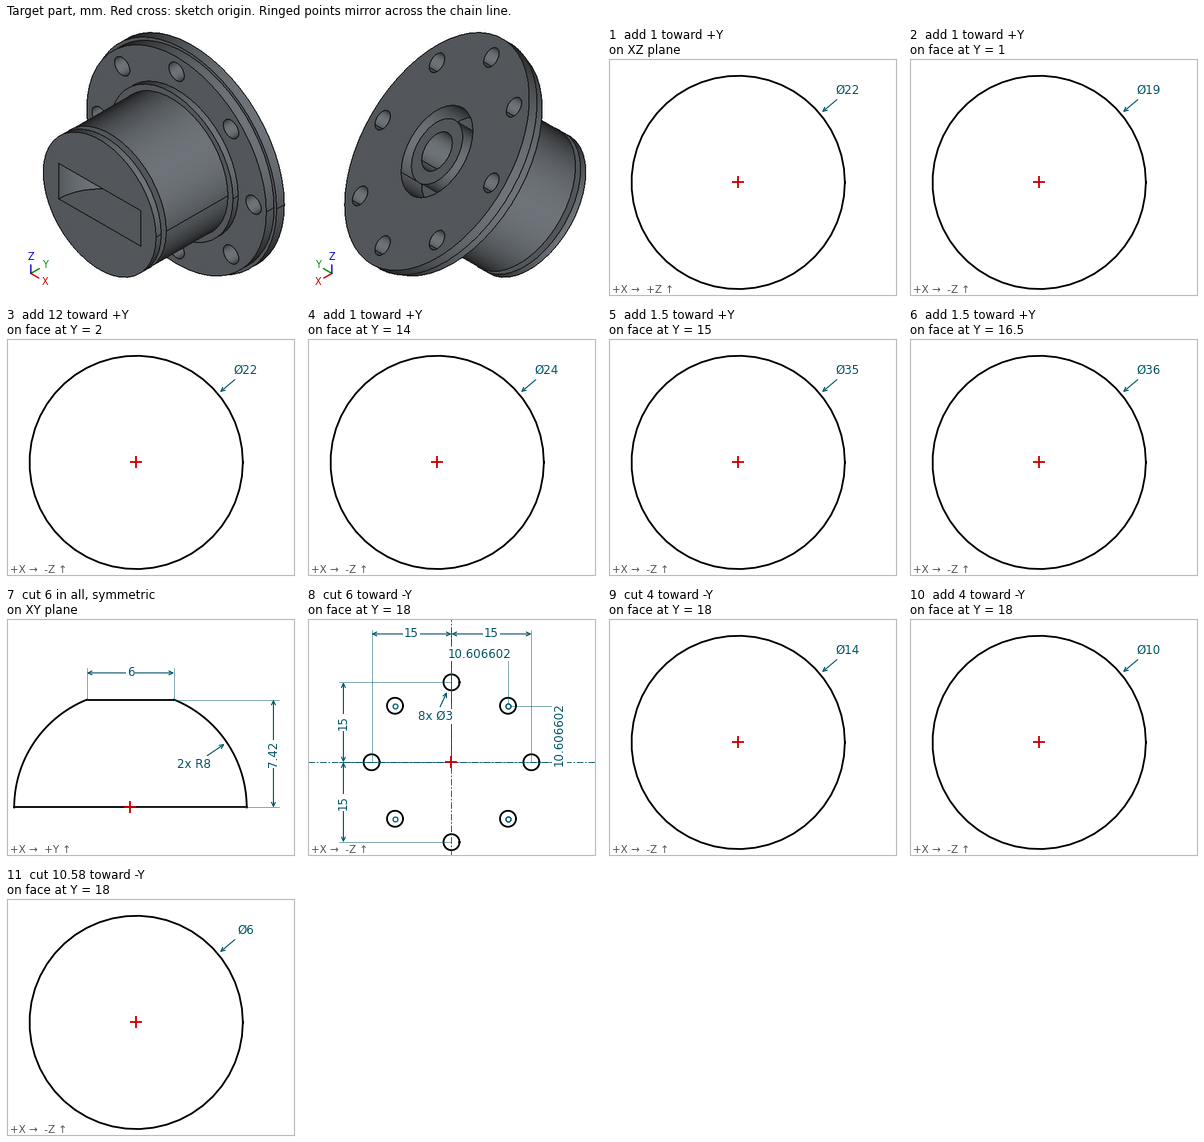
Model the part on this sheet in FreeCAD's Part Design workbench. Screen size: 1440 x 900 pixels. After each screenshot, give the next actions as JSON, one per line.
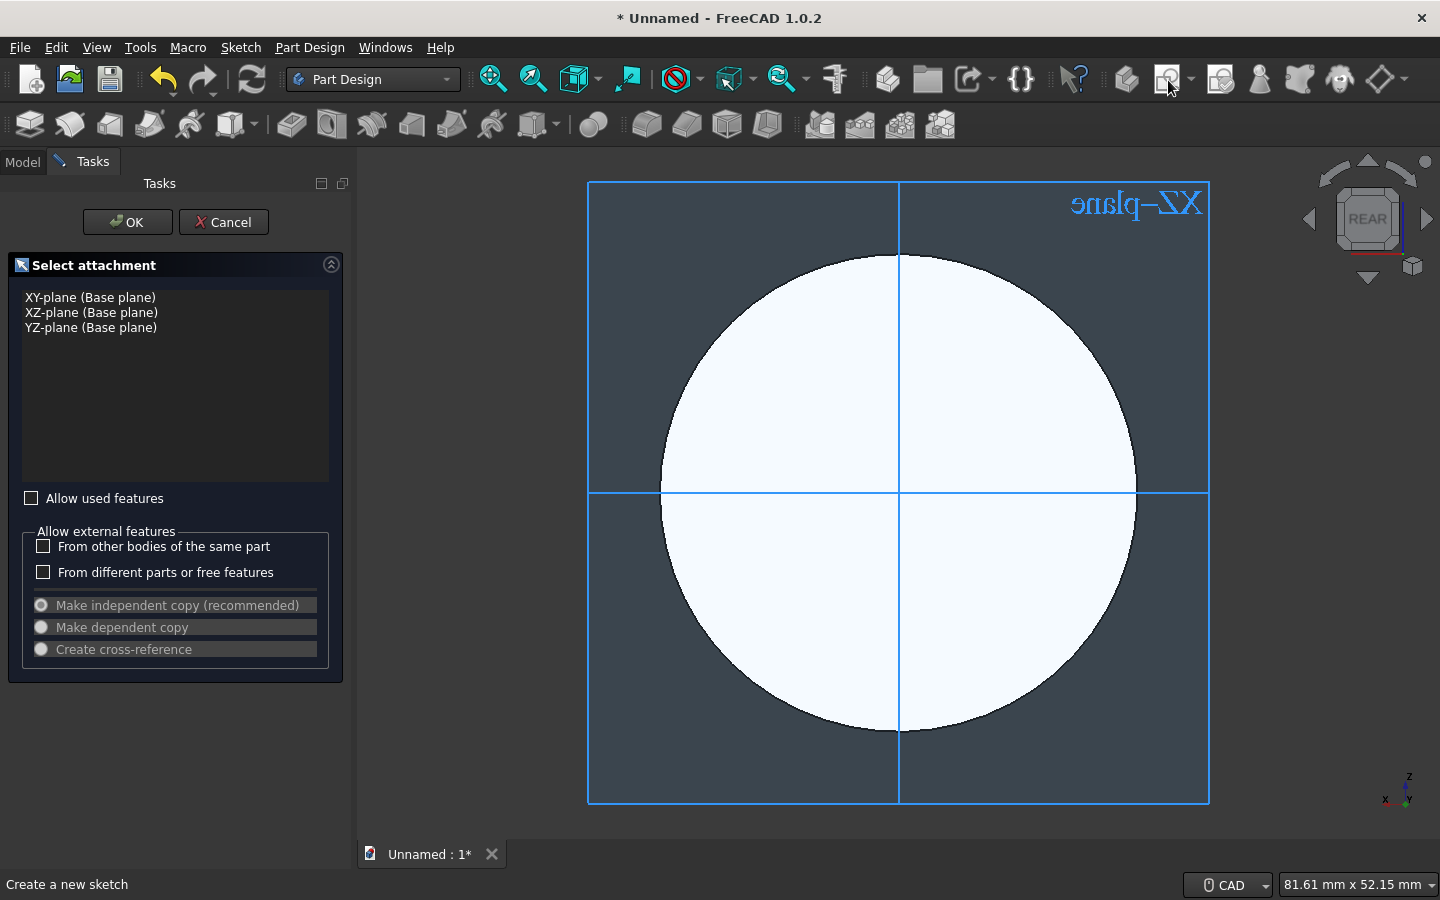
{"action": "left_click", "coordinate": [82, 298]}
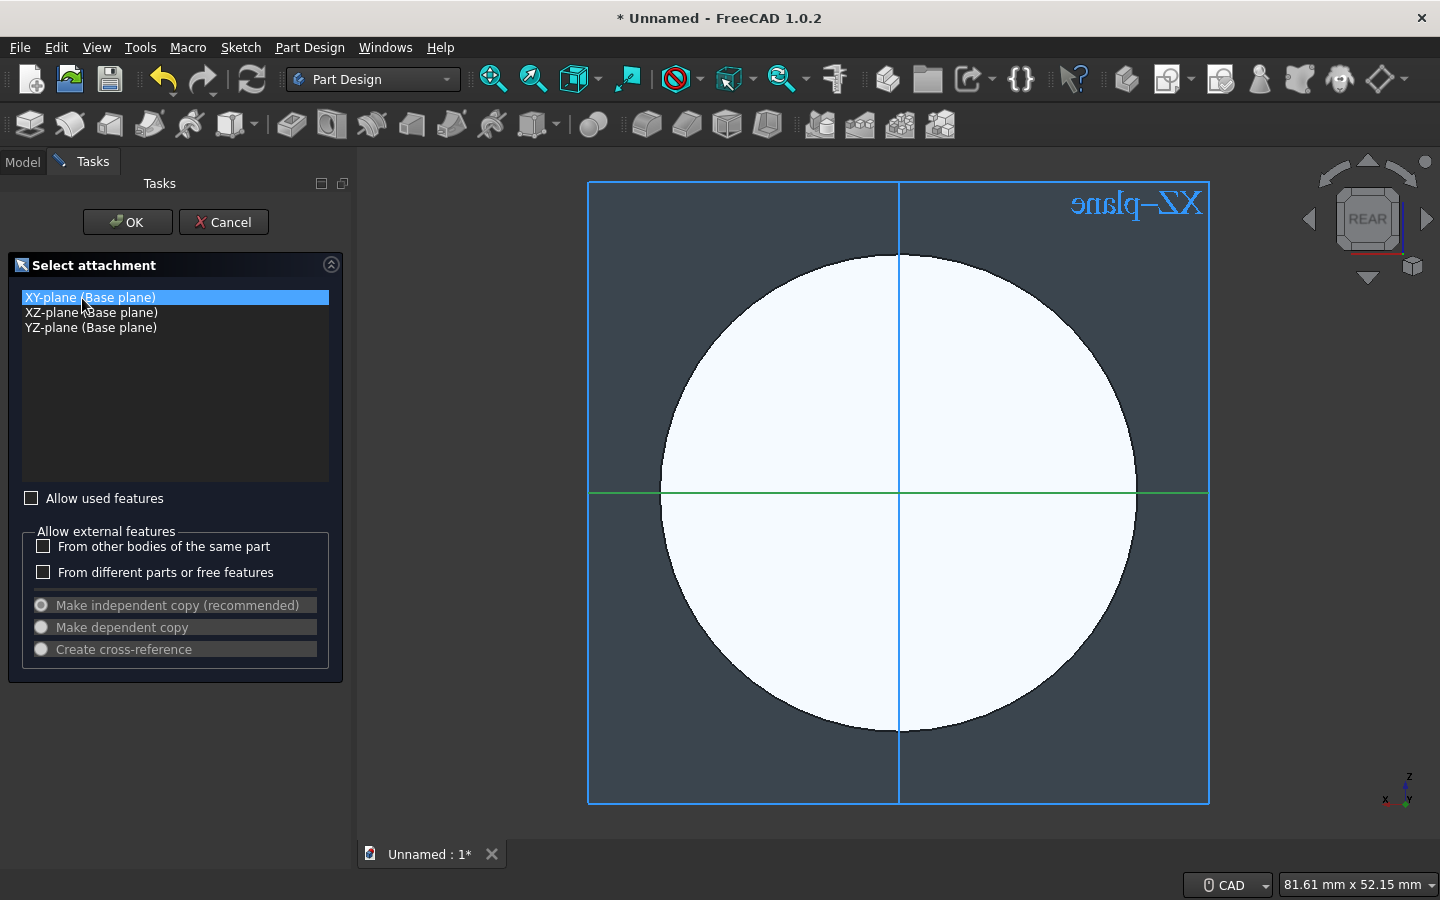
{"action": "left_click", "coordinate": [128, 222]}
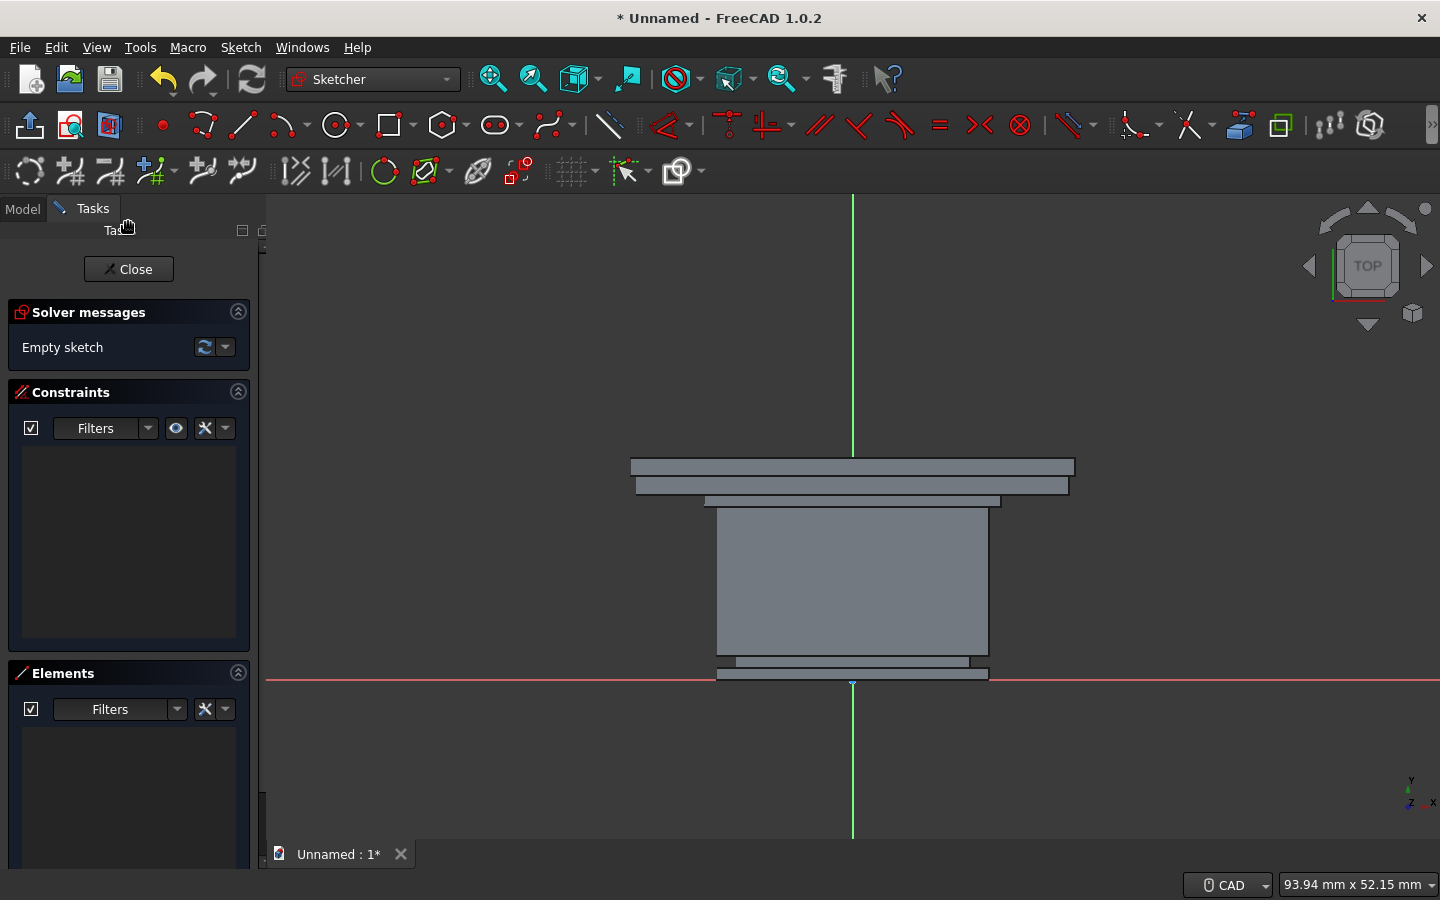
{"action": "left_click", "coordinate": [110, 126]}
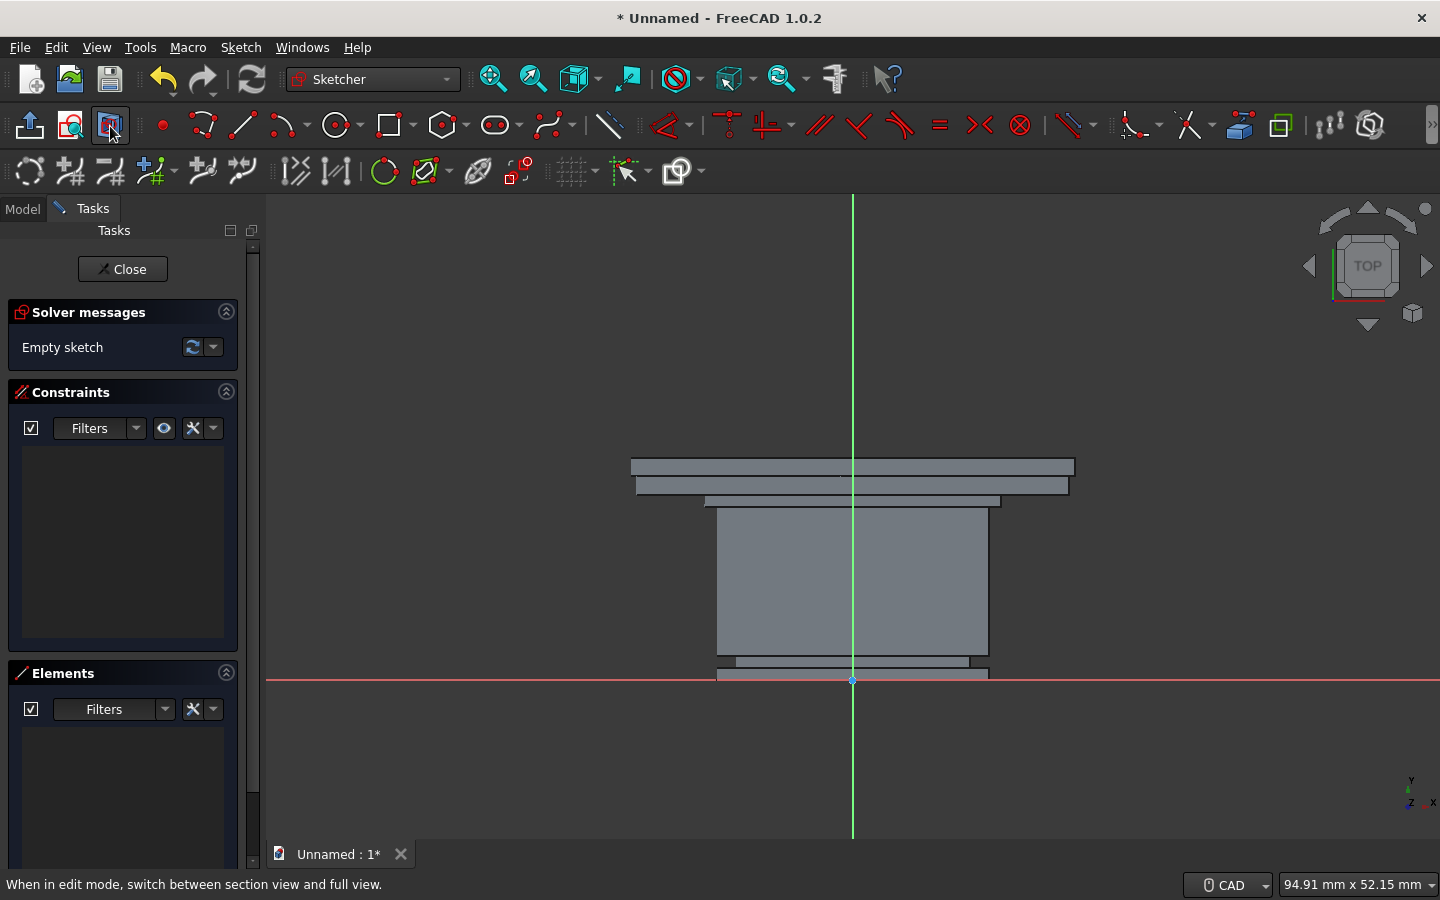
{"action": "scroll", "coordinate": [882, 685], "scroll_direction": "up", "scroll_amount": 6}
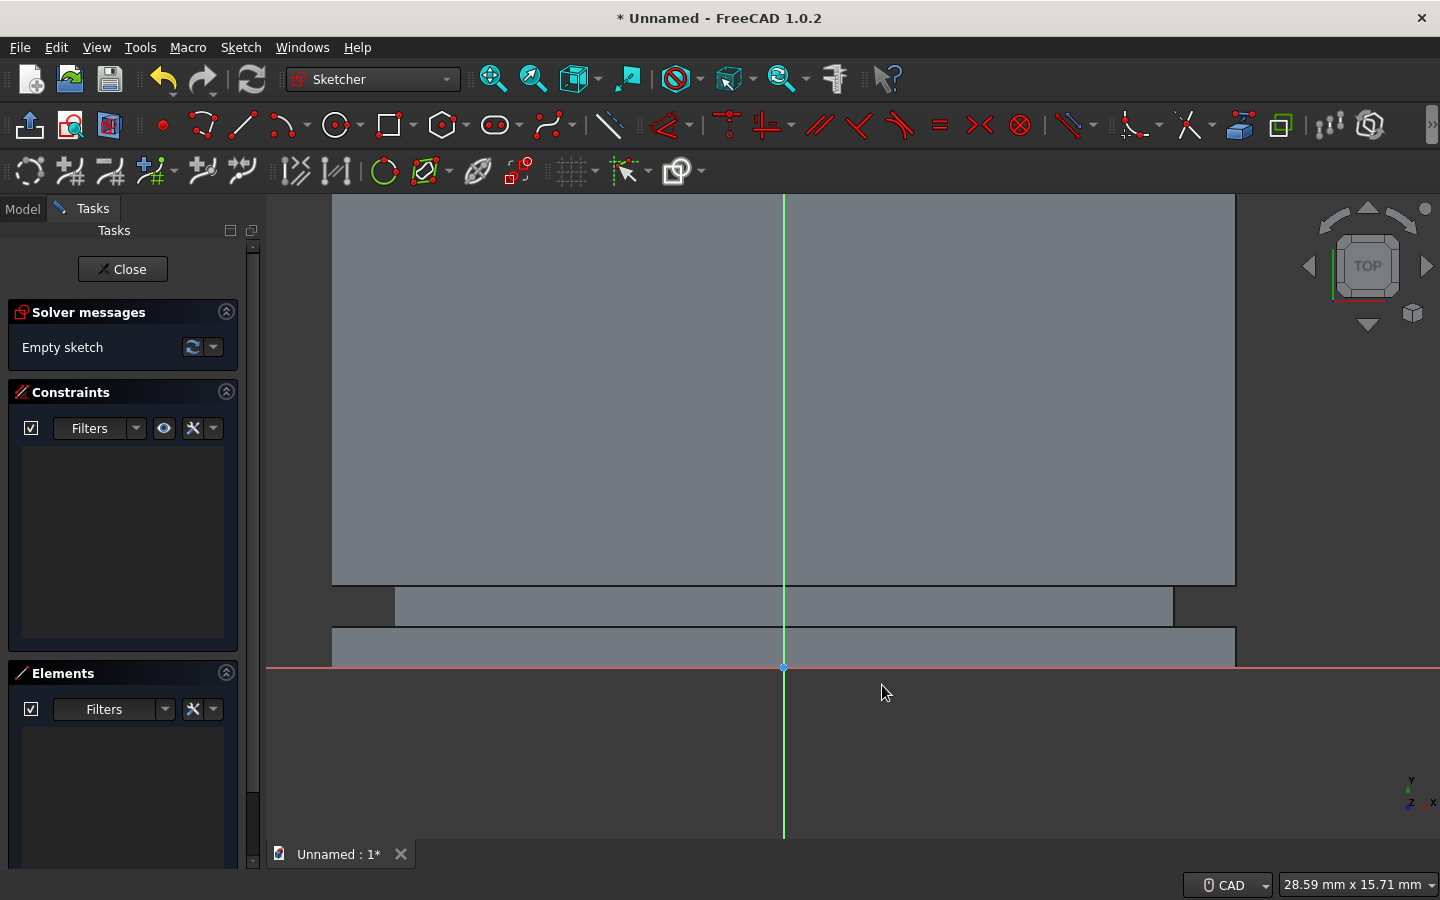
{"action": "left_click", "coordinate": [244, 126]}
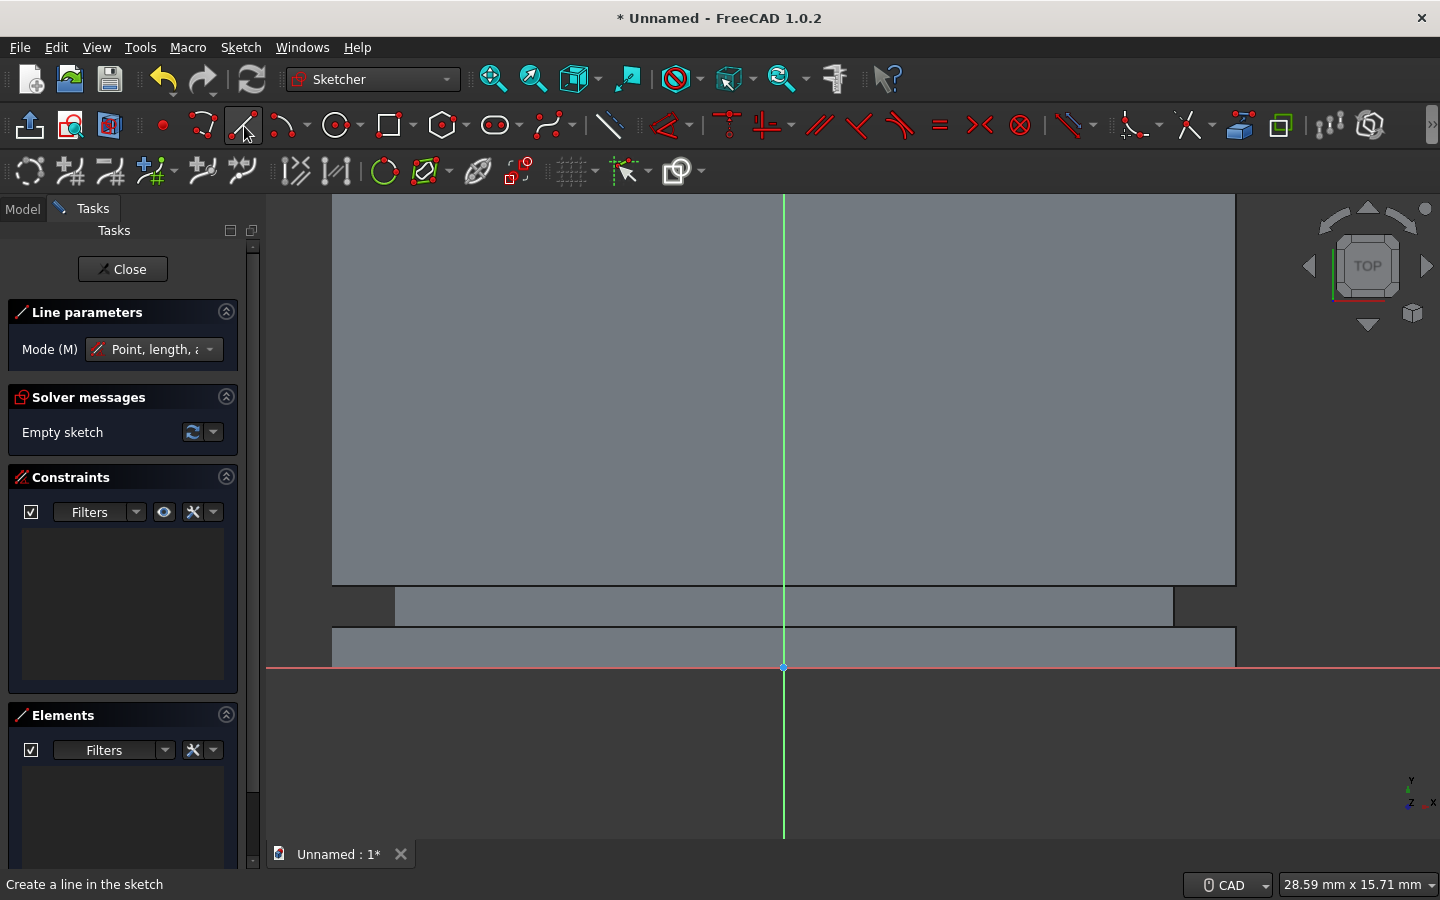
{"action": "left_click", "coordinate": [455, 668]}
{"action": "left_click", "coordinate": [1112, 659]}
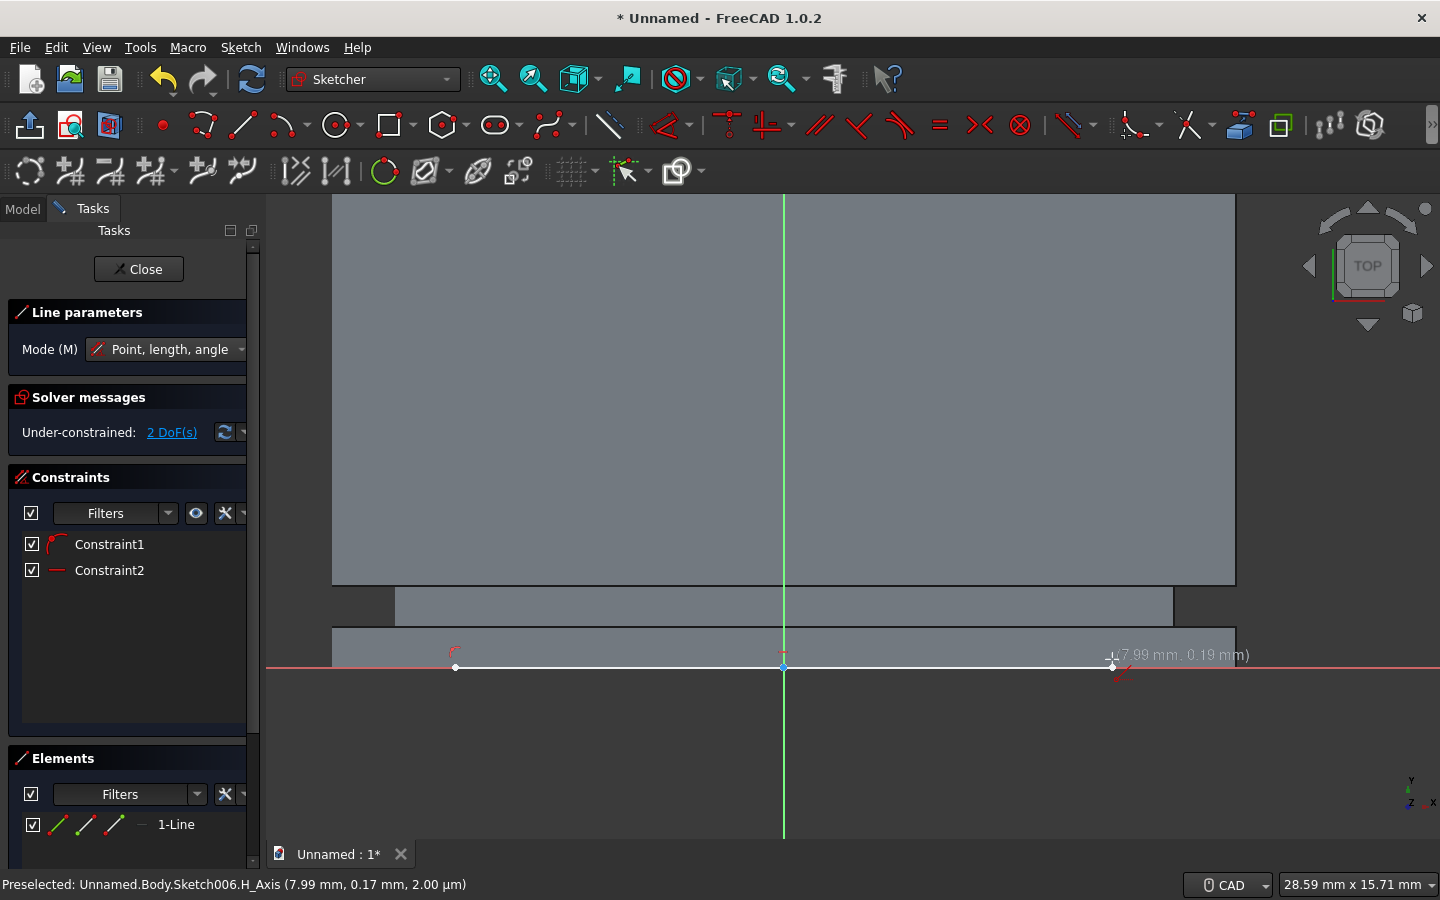
{"action": "left_click", "coordinate": [907, 363]}
{"action": "left_click", "coordinate": [661, 363]}